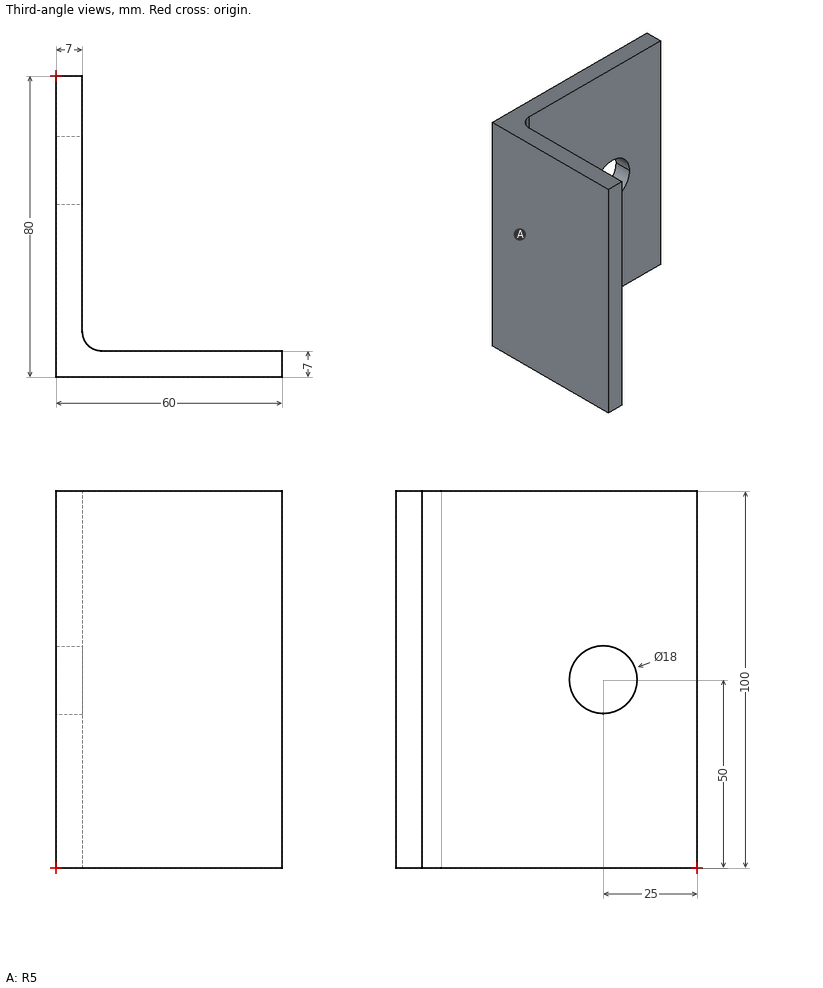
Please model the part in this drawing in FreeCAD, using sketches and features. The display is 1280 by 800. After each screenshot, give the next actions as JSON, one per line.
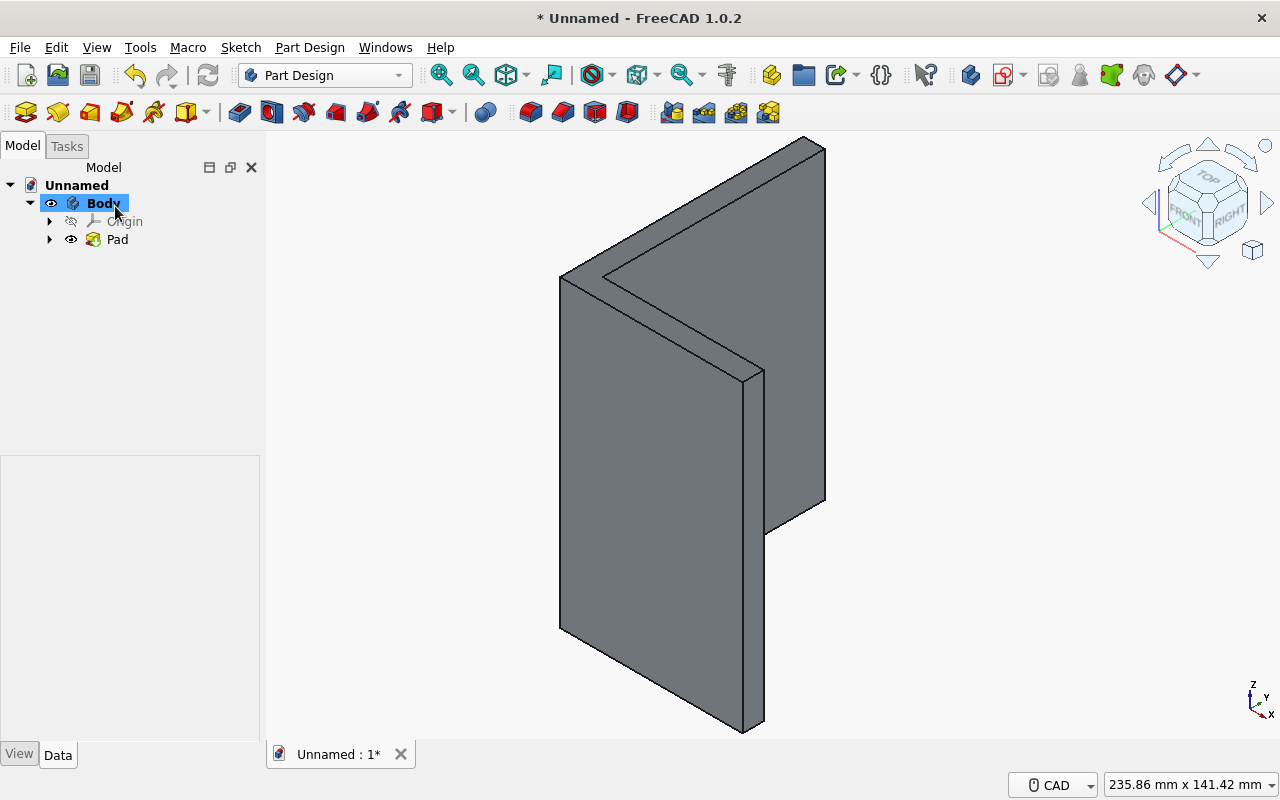
{"action": "left_click", "coordinate": [745, 319]}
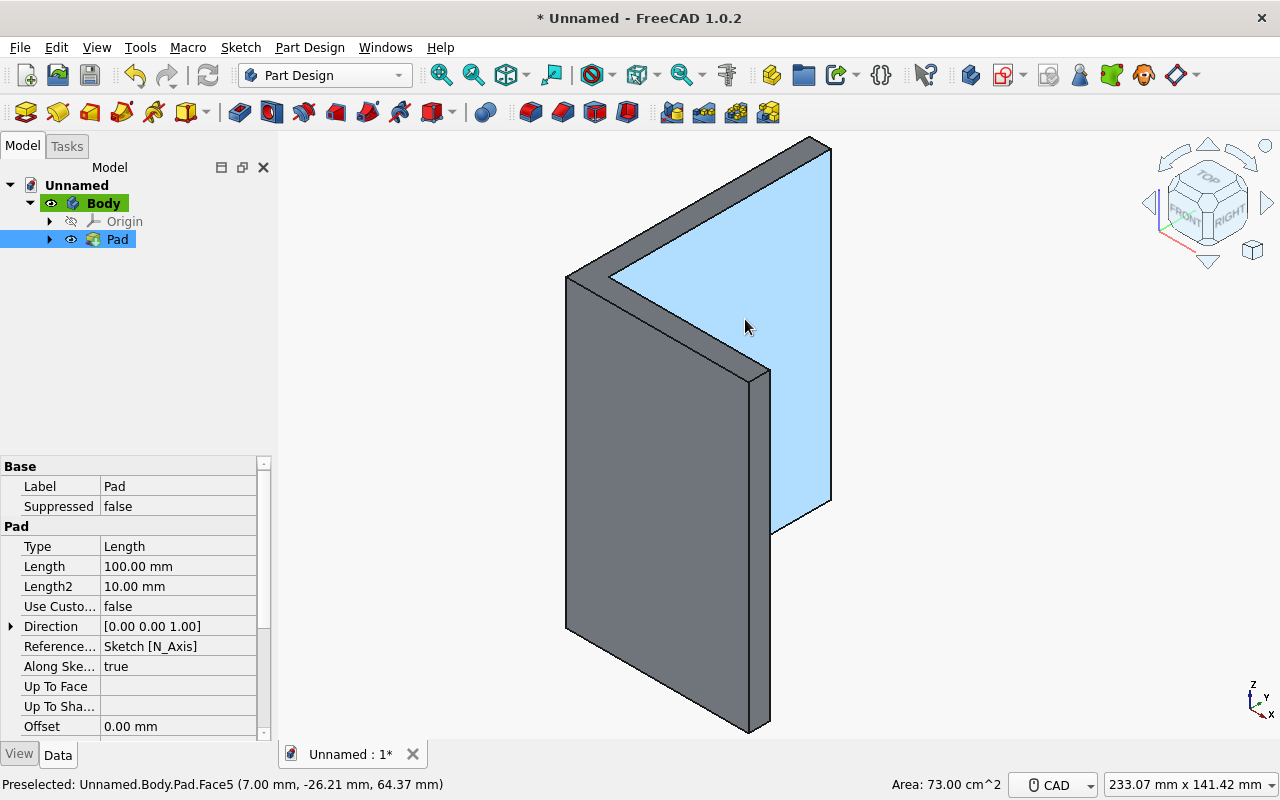
{"action": "left_click", "coordinate": [1004, 76]}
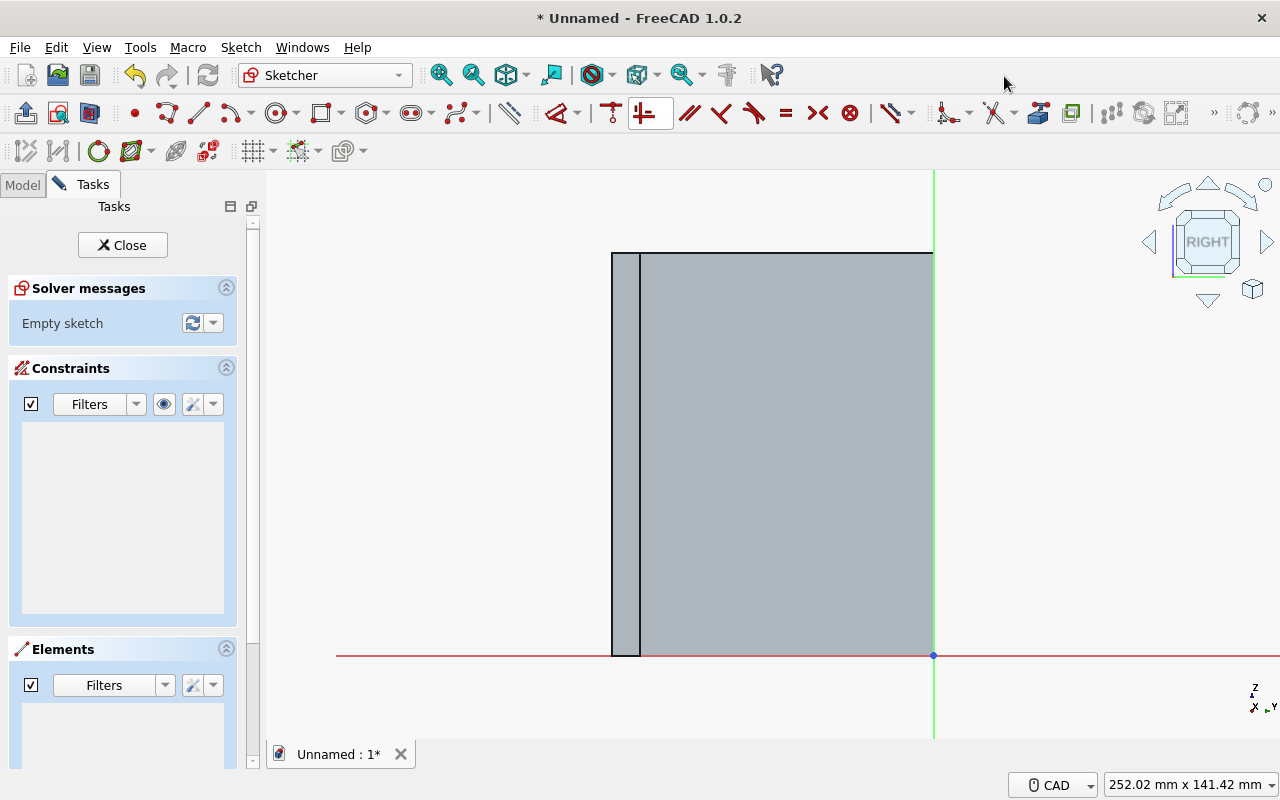
{"action": "scroll", "coordinate": [866, 454], "scroll_direction": "up", "scroll_amount": 8}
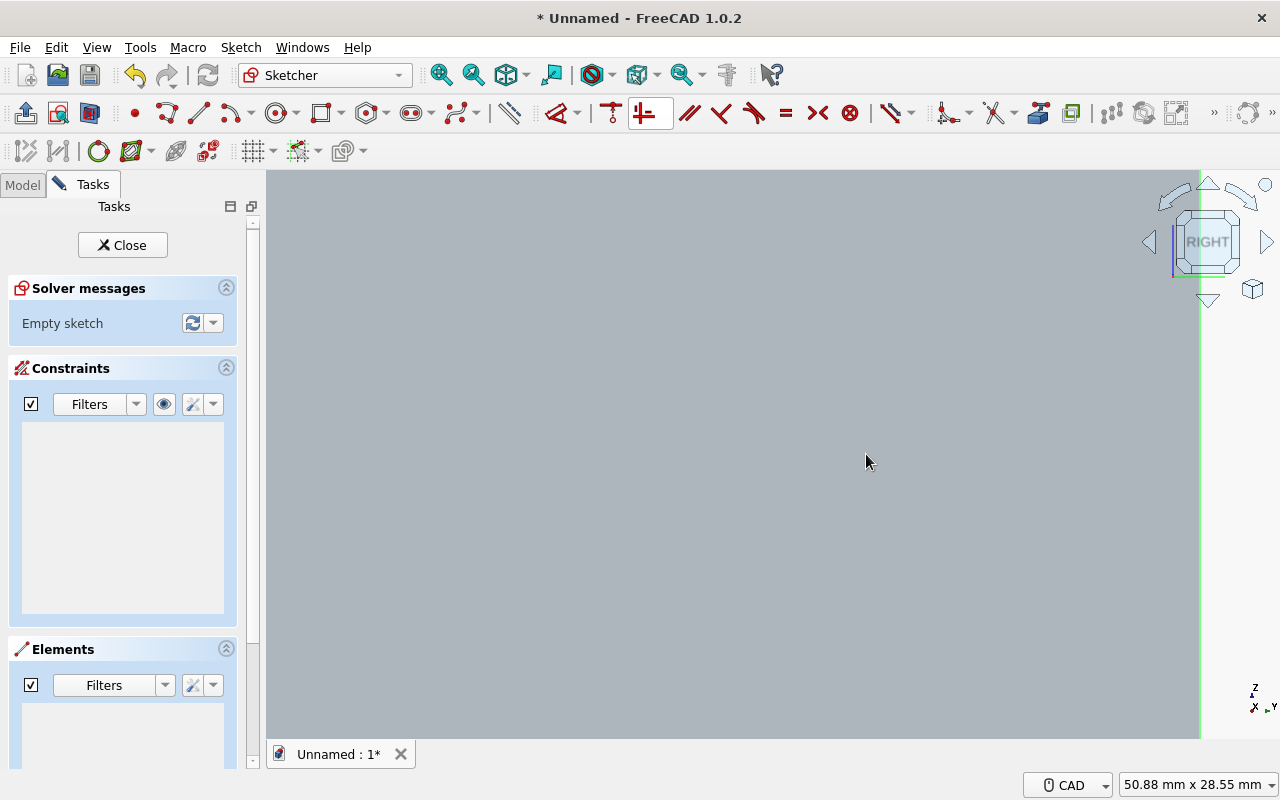
{"action": "key", "text": "g c"}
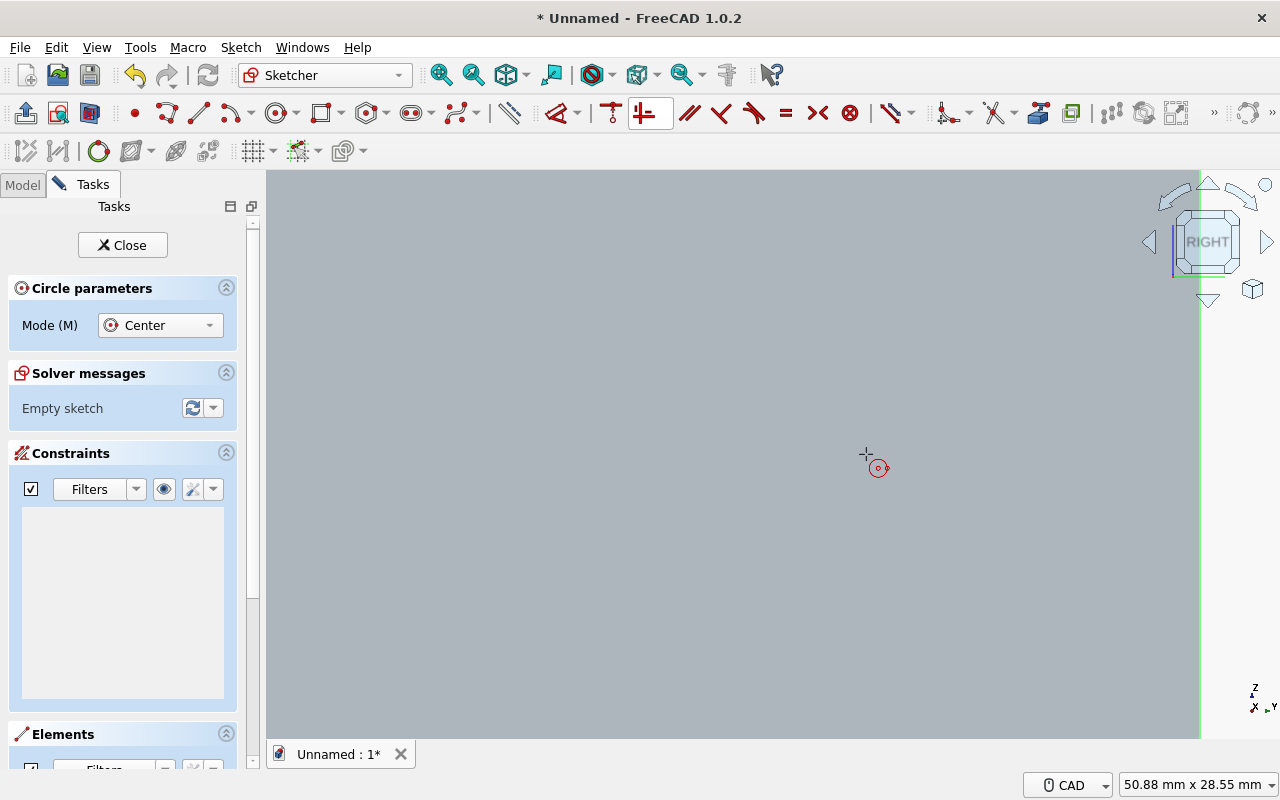
{"action": "left_click", "coordinate": [702, 454]}
{"action": "left_click", "coordinate": [829, 328]}
{"action": "key", "text": "Escape"}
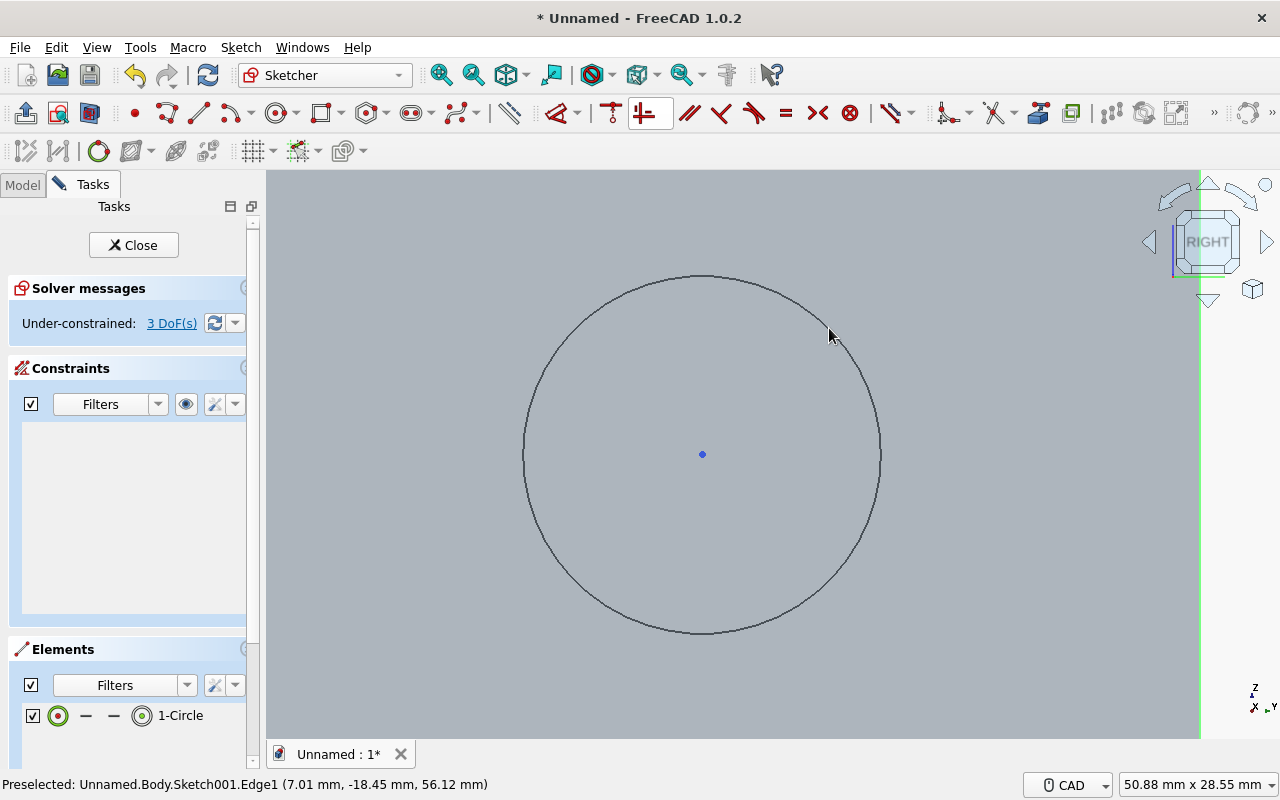
{"action": "left_click", "coordinate": [556, 114]}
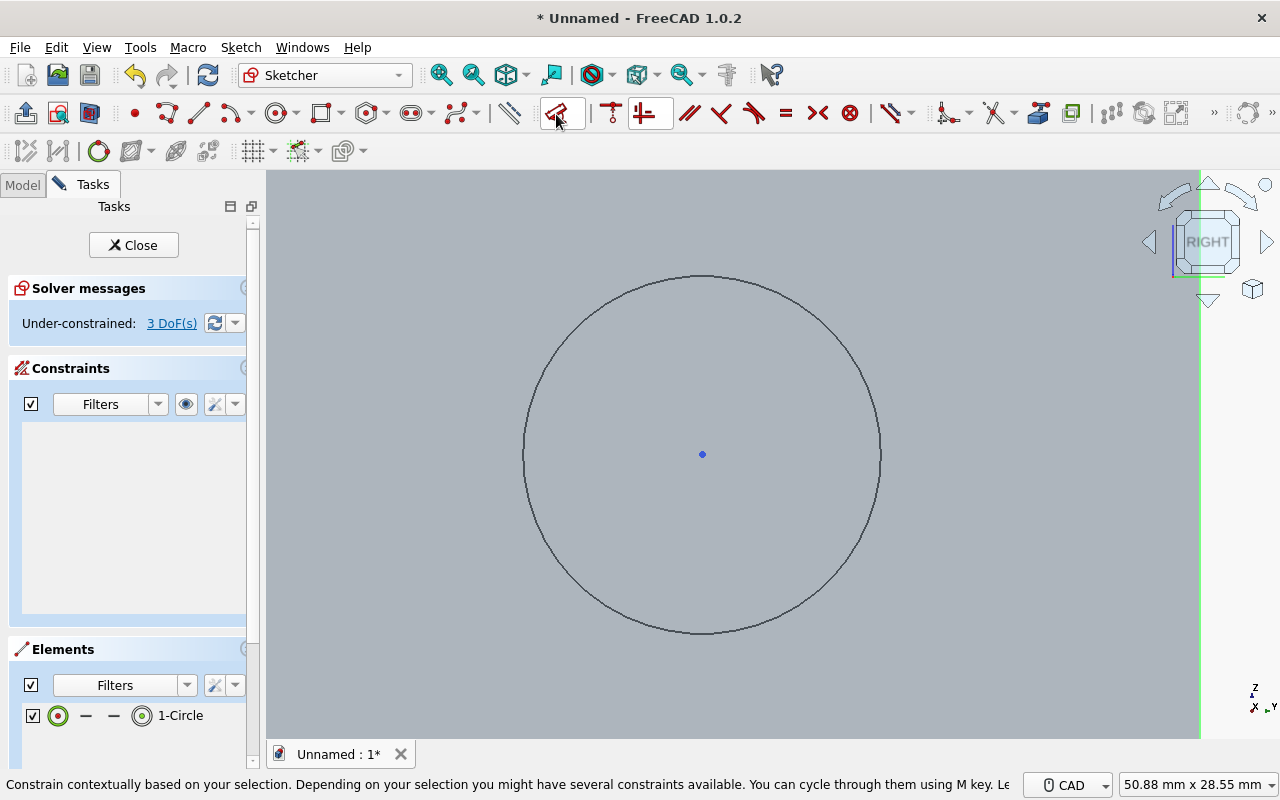
{"action": "left_click", "coordinate": [828, 328]}
{"action": "left_click", "coordinate": [851, 305]}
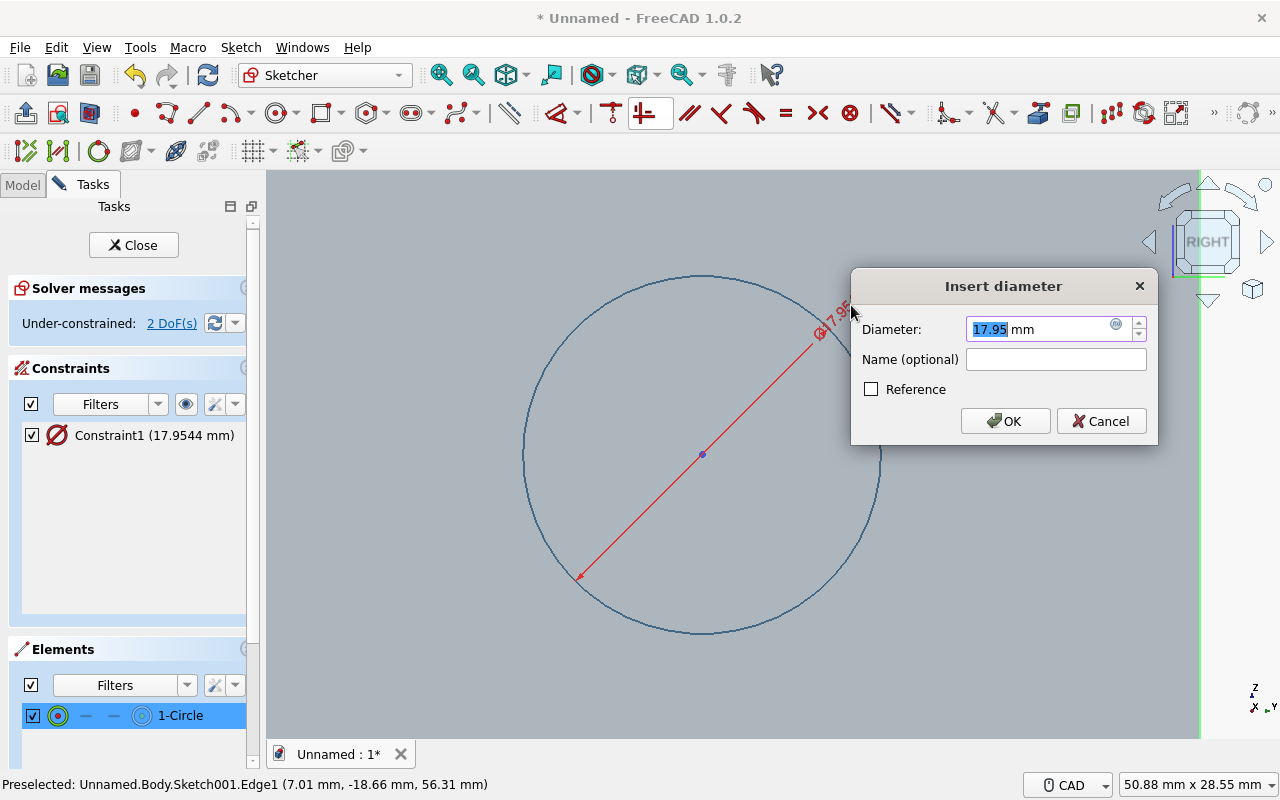
{"action": "type", "text": "18"}
{"action": "key", "text": "Return"}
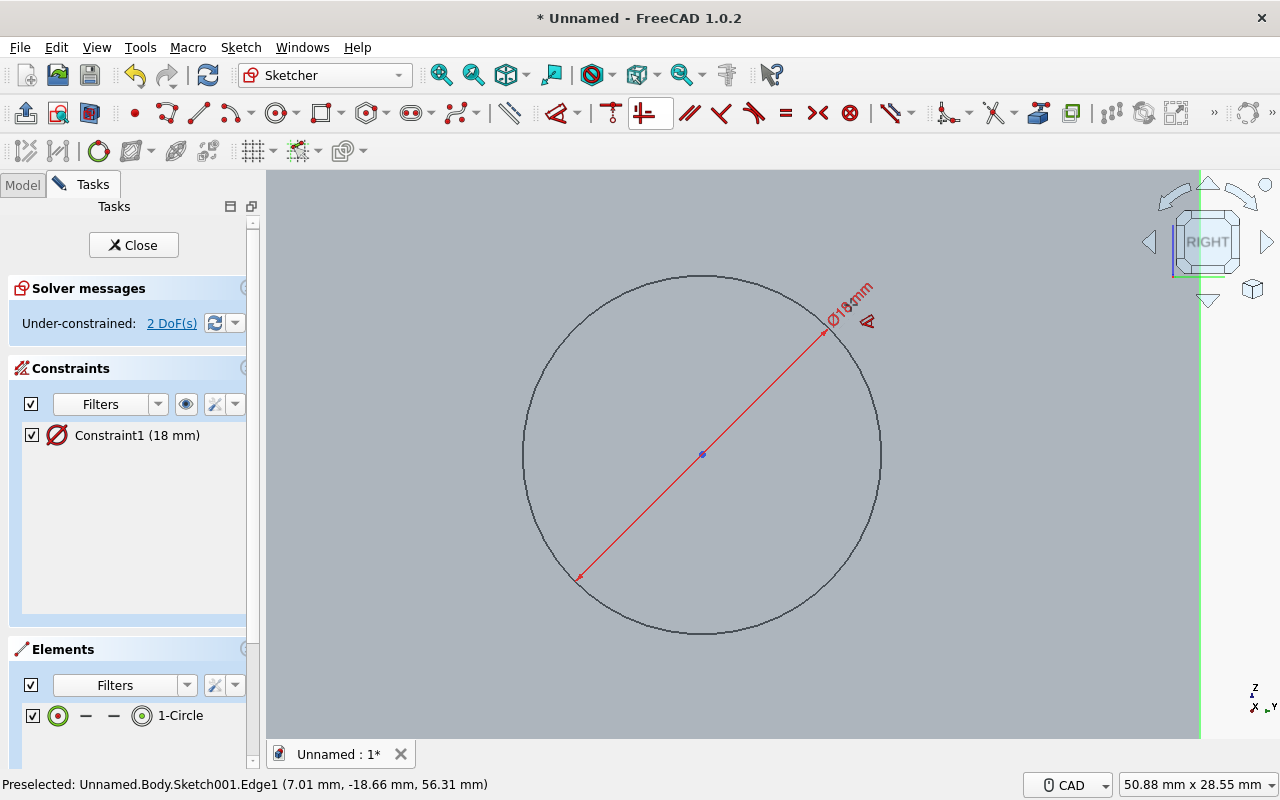
{"action": "left_click", "coordinate": [702, 455]}
{"action": "left_click", "coordinate": [908, 421]}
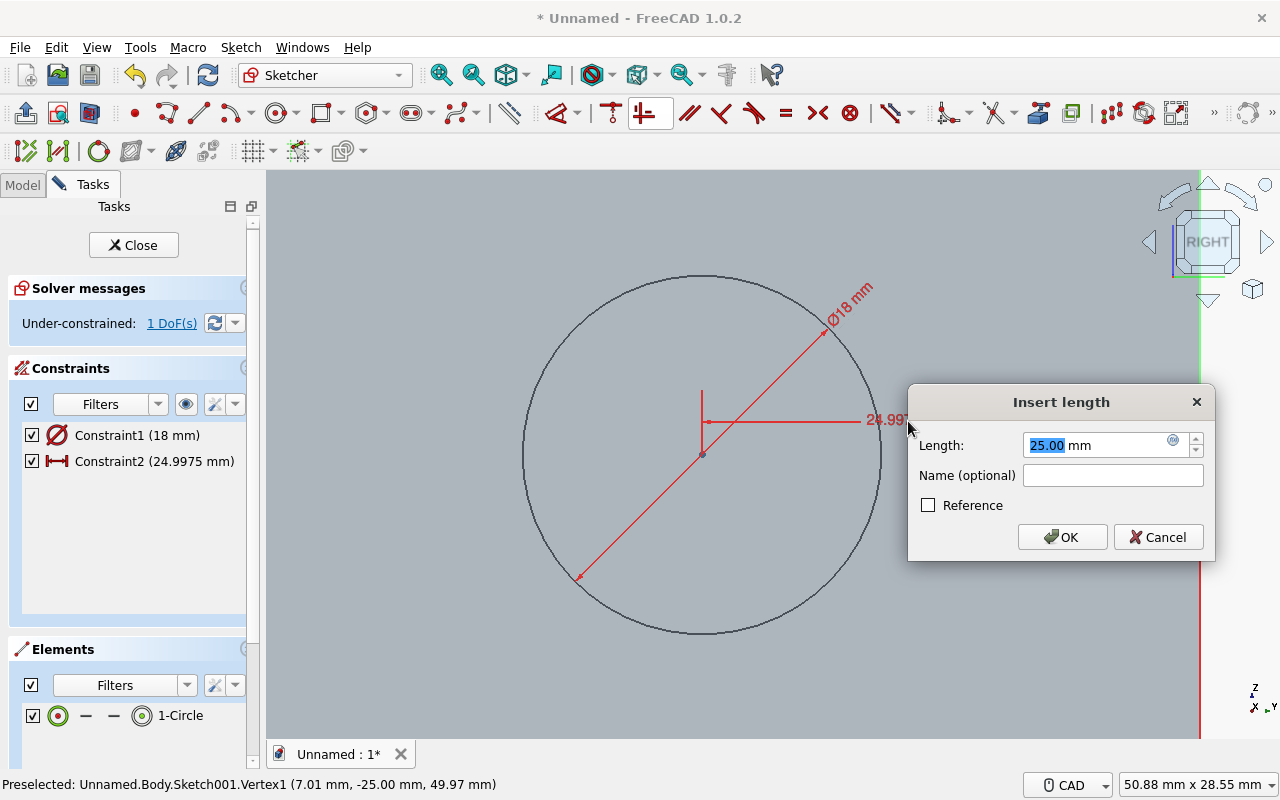
{"action": "type", "text": "25"}
{"action": "key", "text": "Return"}